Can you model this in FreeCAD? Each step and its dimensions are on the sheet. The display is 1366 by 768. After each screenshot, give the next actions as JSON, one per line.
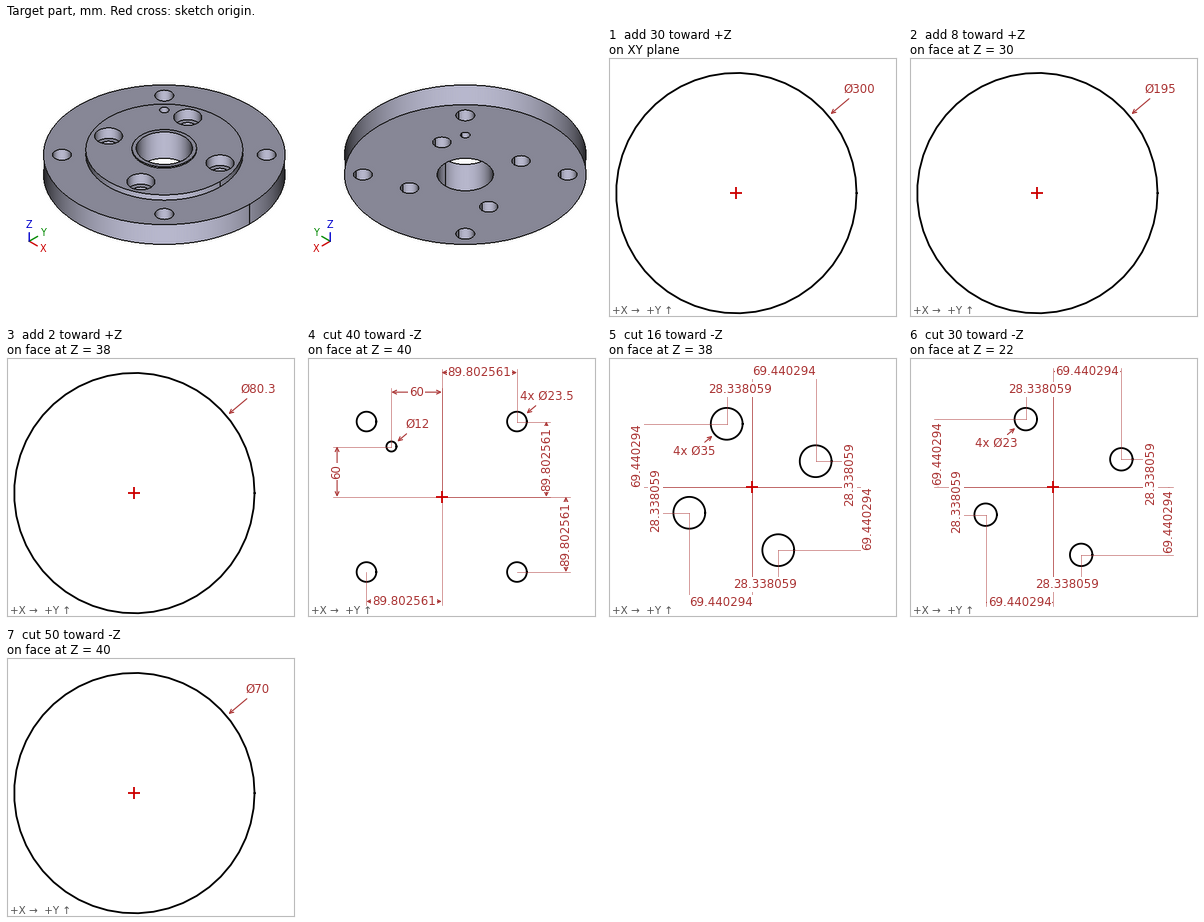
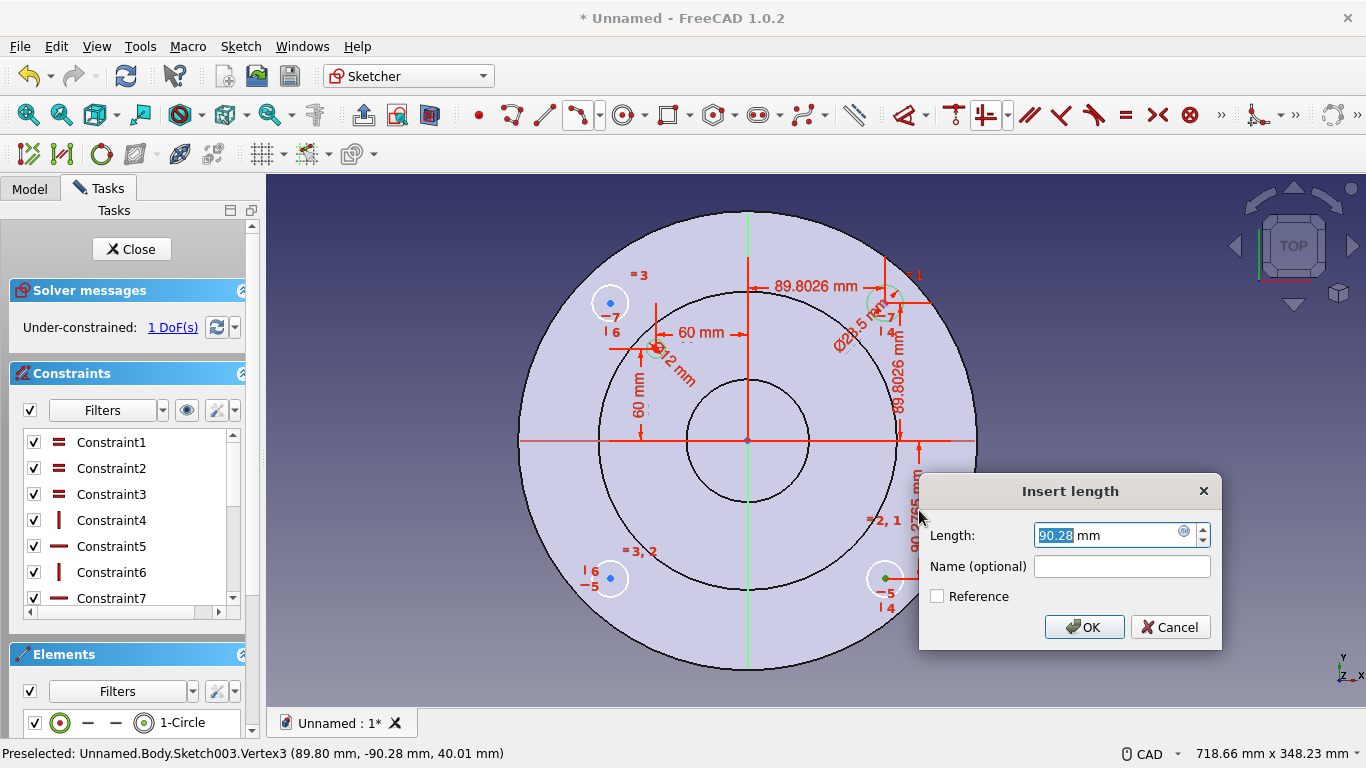
{"action": "type", "text": "89.802561"}
{"action": "key", "text": "Return"}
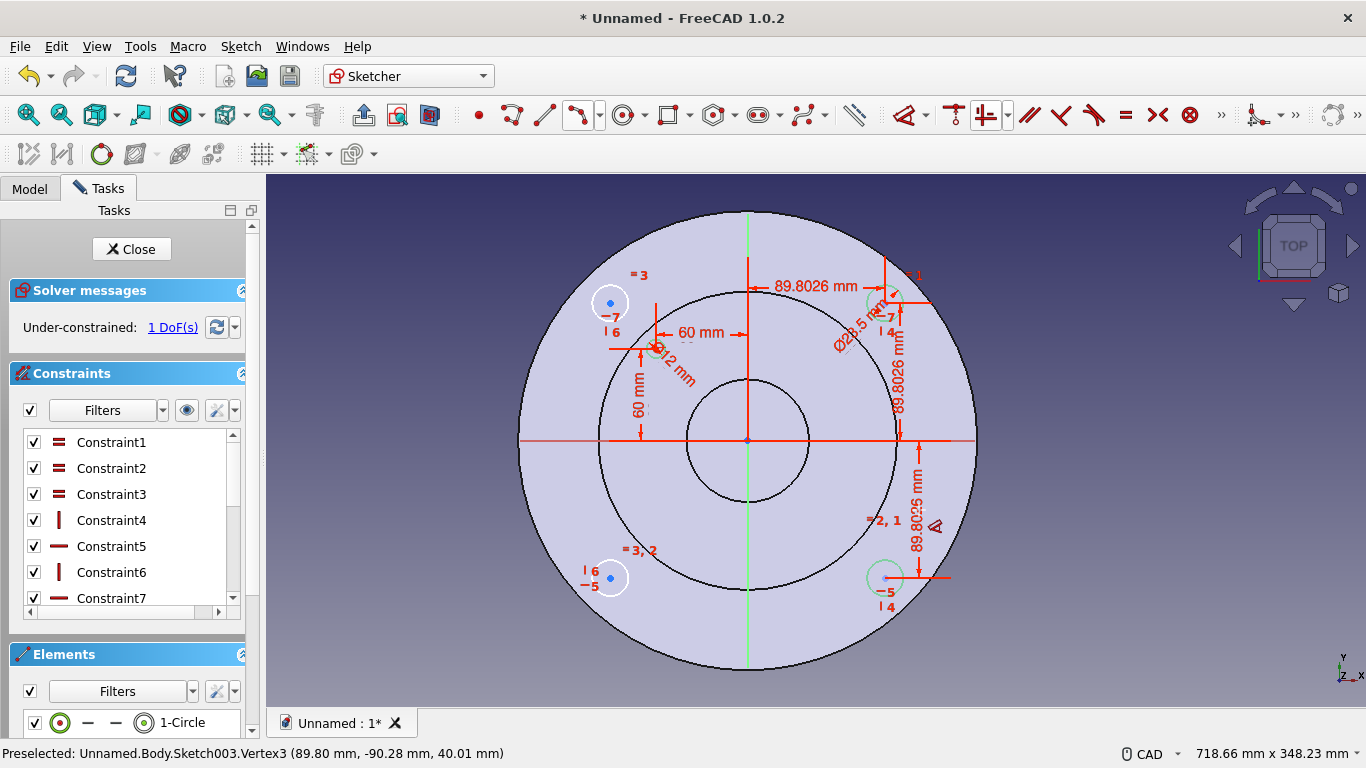
{"action": "left_click", "coordinate": [610, 578]}
{"action": "left_click", "coordinate": [679, 612]}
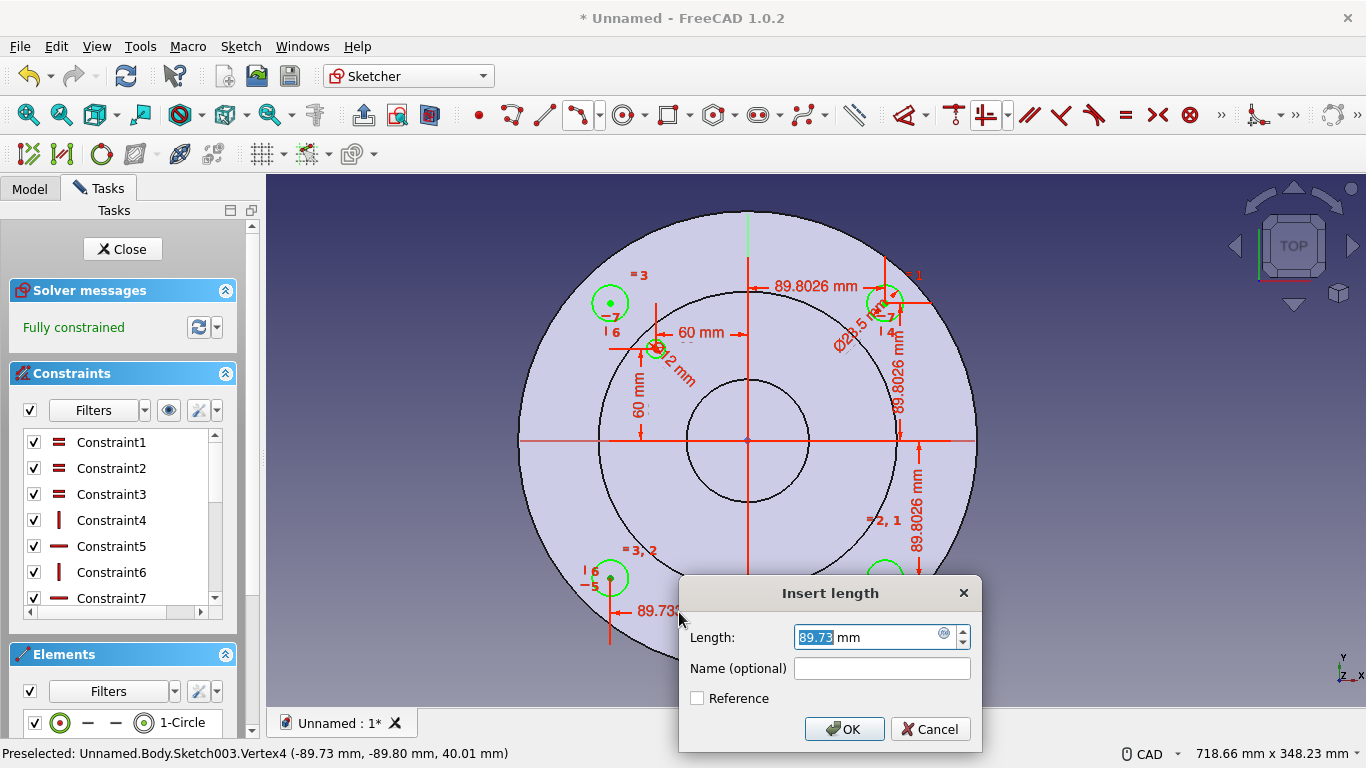
{"action": "type", "text": "89.802561"}
{"action": "key", "text": "Return"}
{"action": "key", "text": "Escape"}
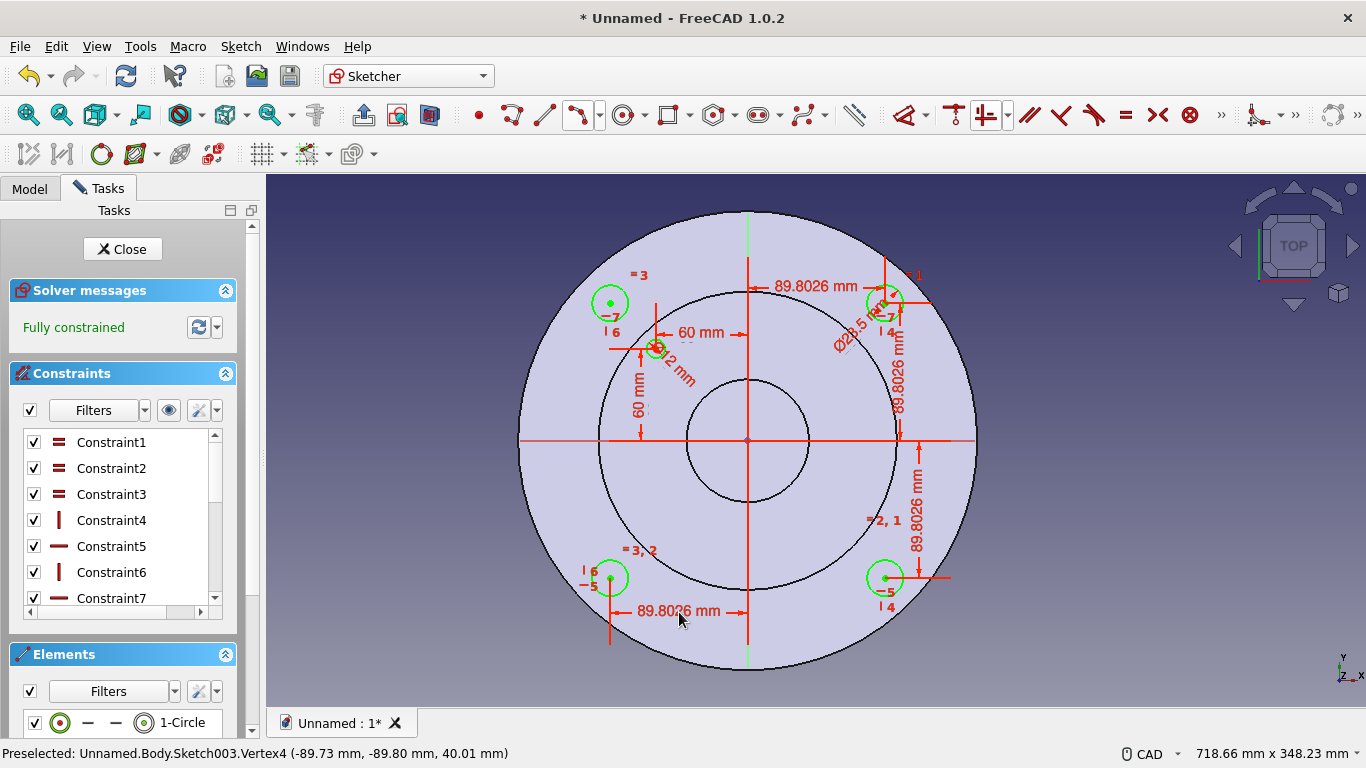
{"action": "left_click", "coordinate": [123, 249]}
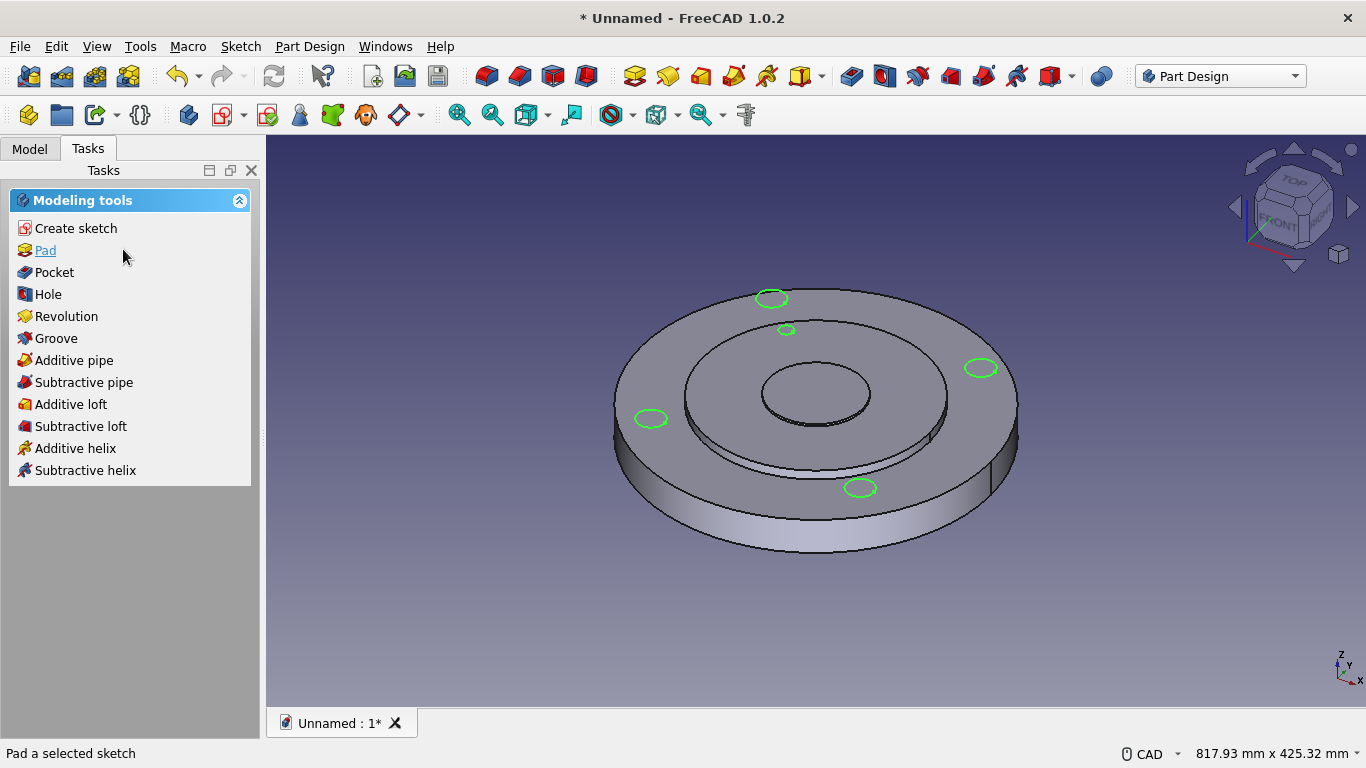
{"action": "left_click", "coordinate": [852, 76]}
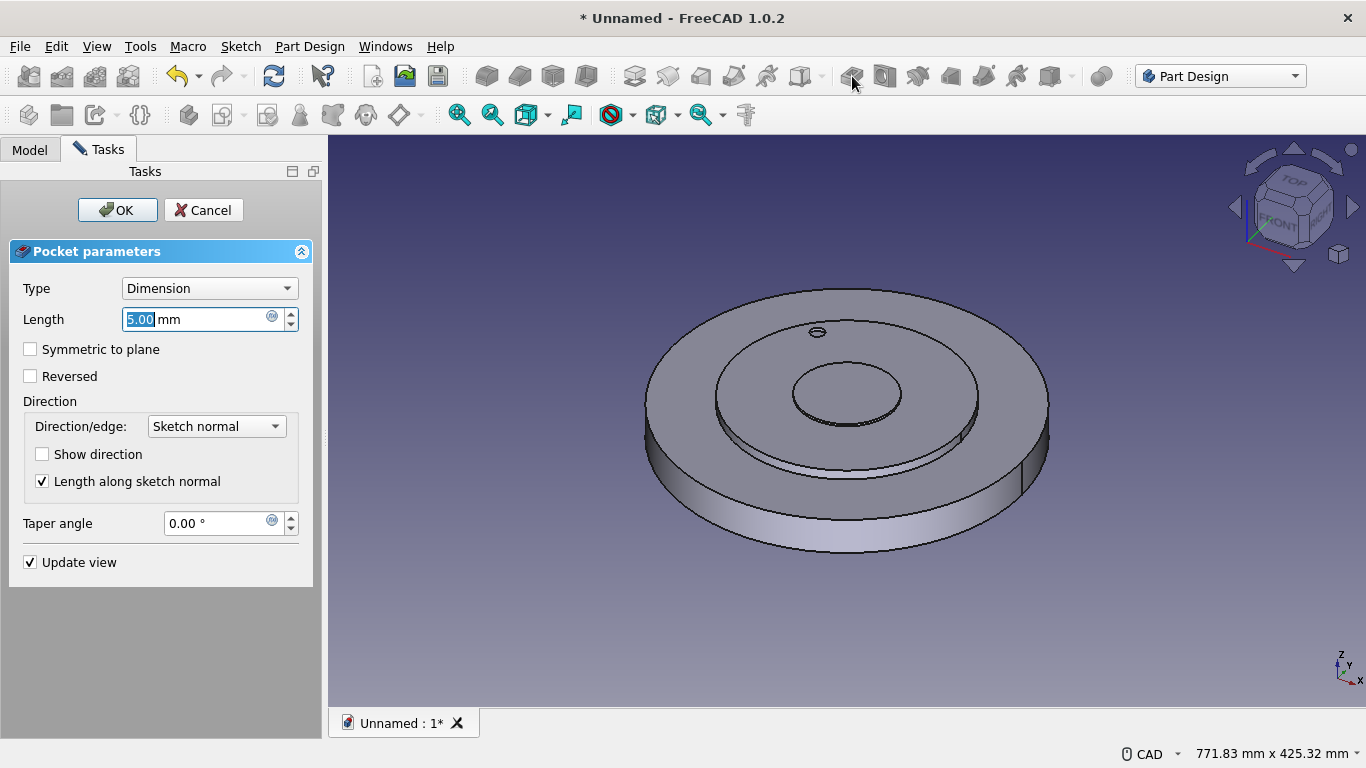
{"action": "type", "text": "40"}
{"action": "key", "text": "Tab"}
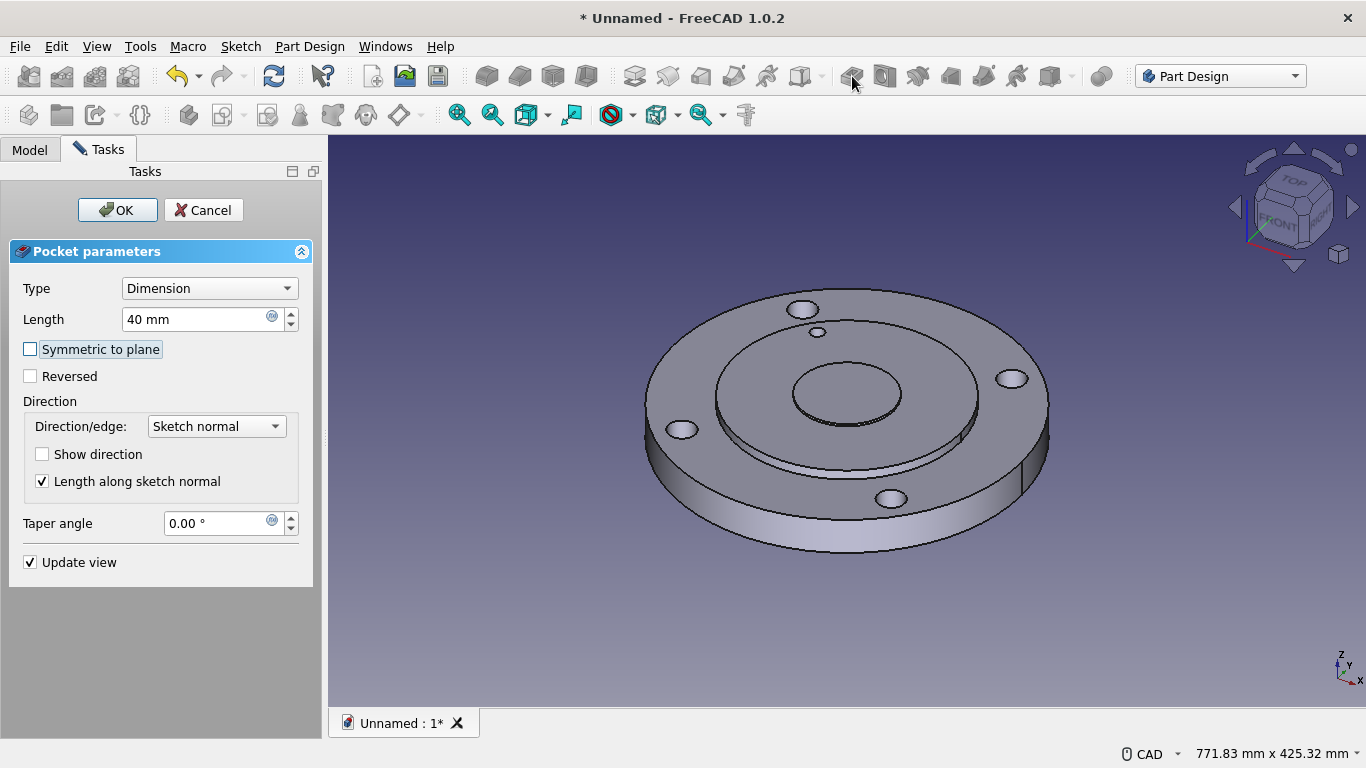
{"action": "left_click", "coordinate": [118, 210]}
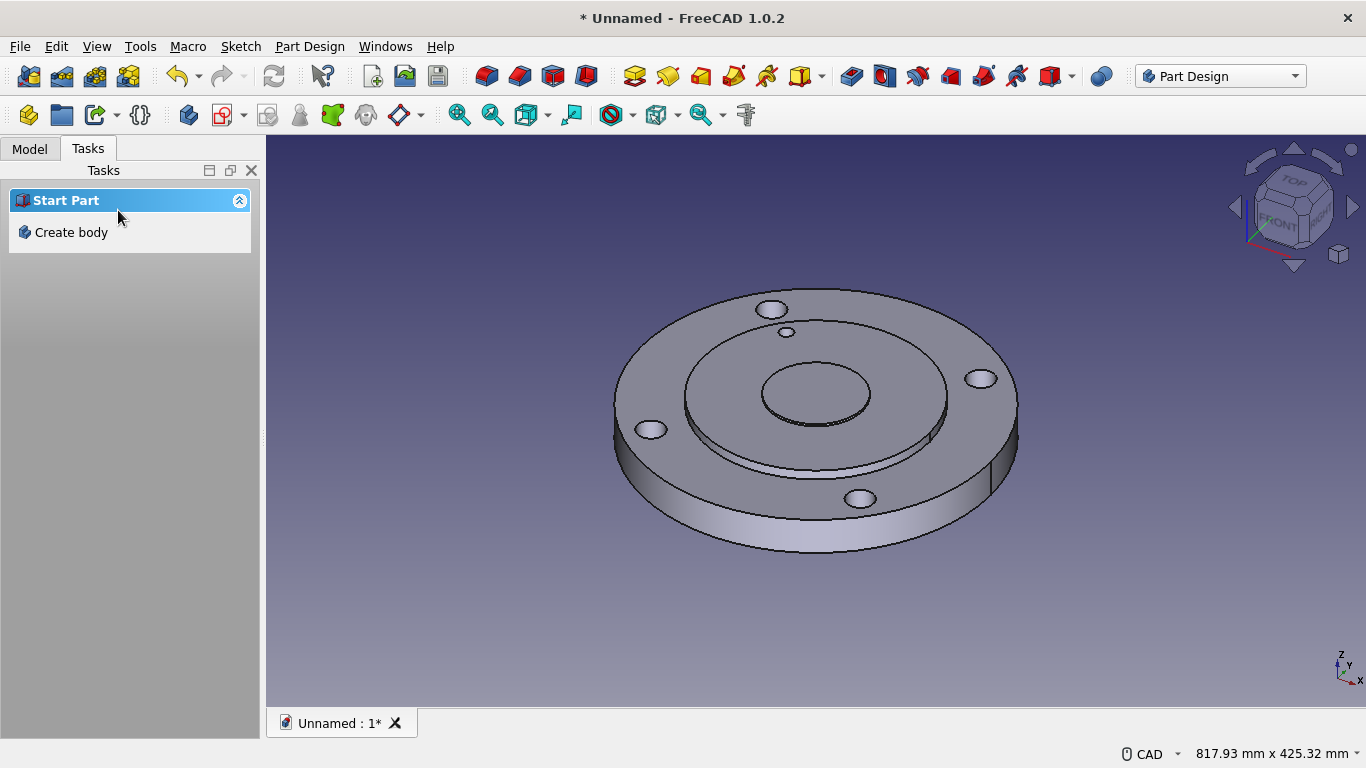
{"action": "left_click", "coordinate": [900, 397]}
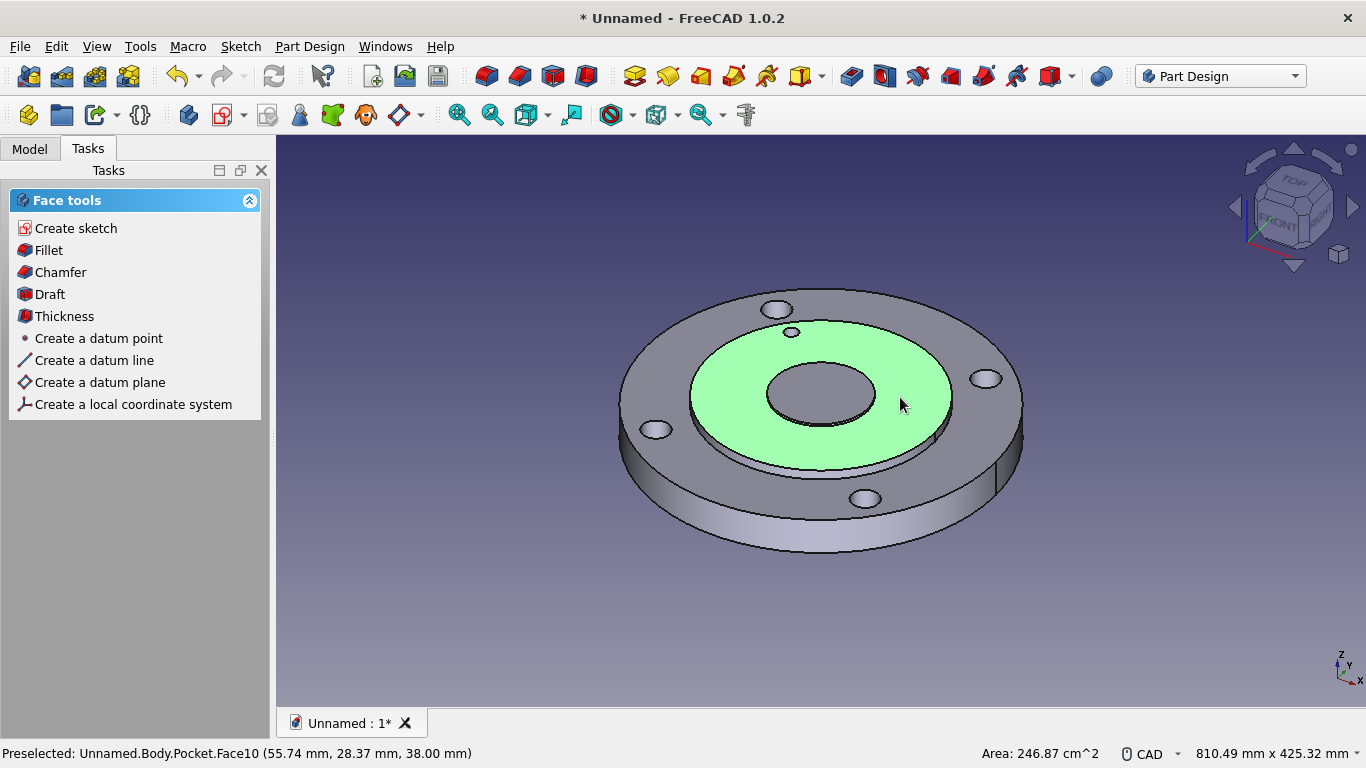
{"action": "left_click", "coordinate": [222, 116]}